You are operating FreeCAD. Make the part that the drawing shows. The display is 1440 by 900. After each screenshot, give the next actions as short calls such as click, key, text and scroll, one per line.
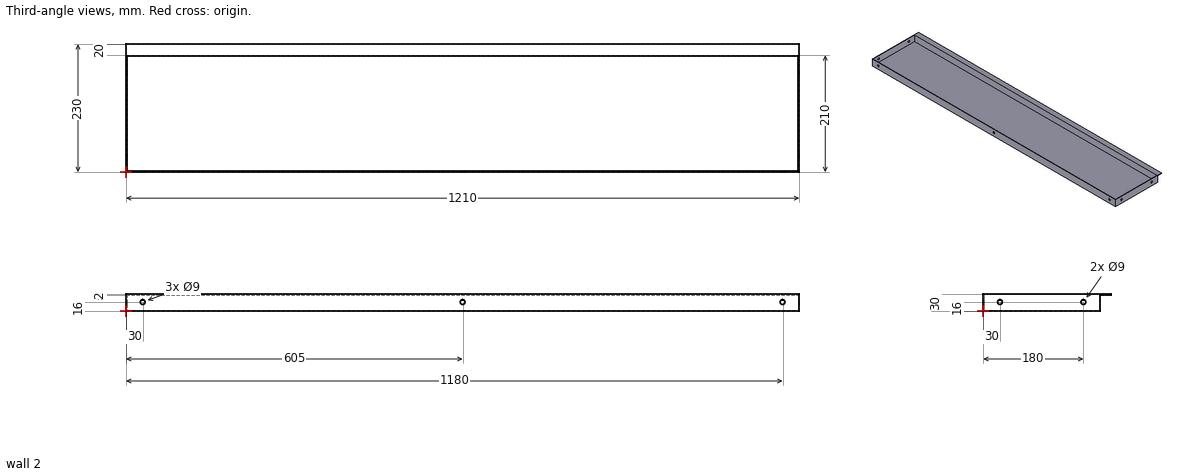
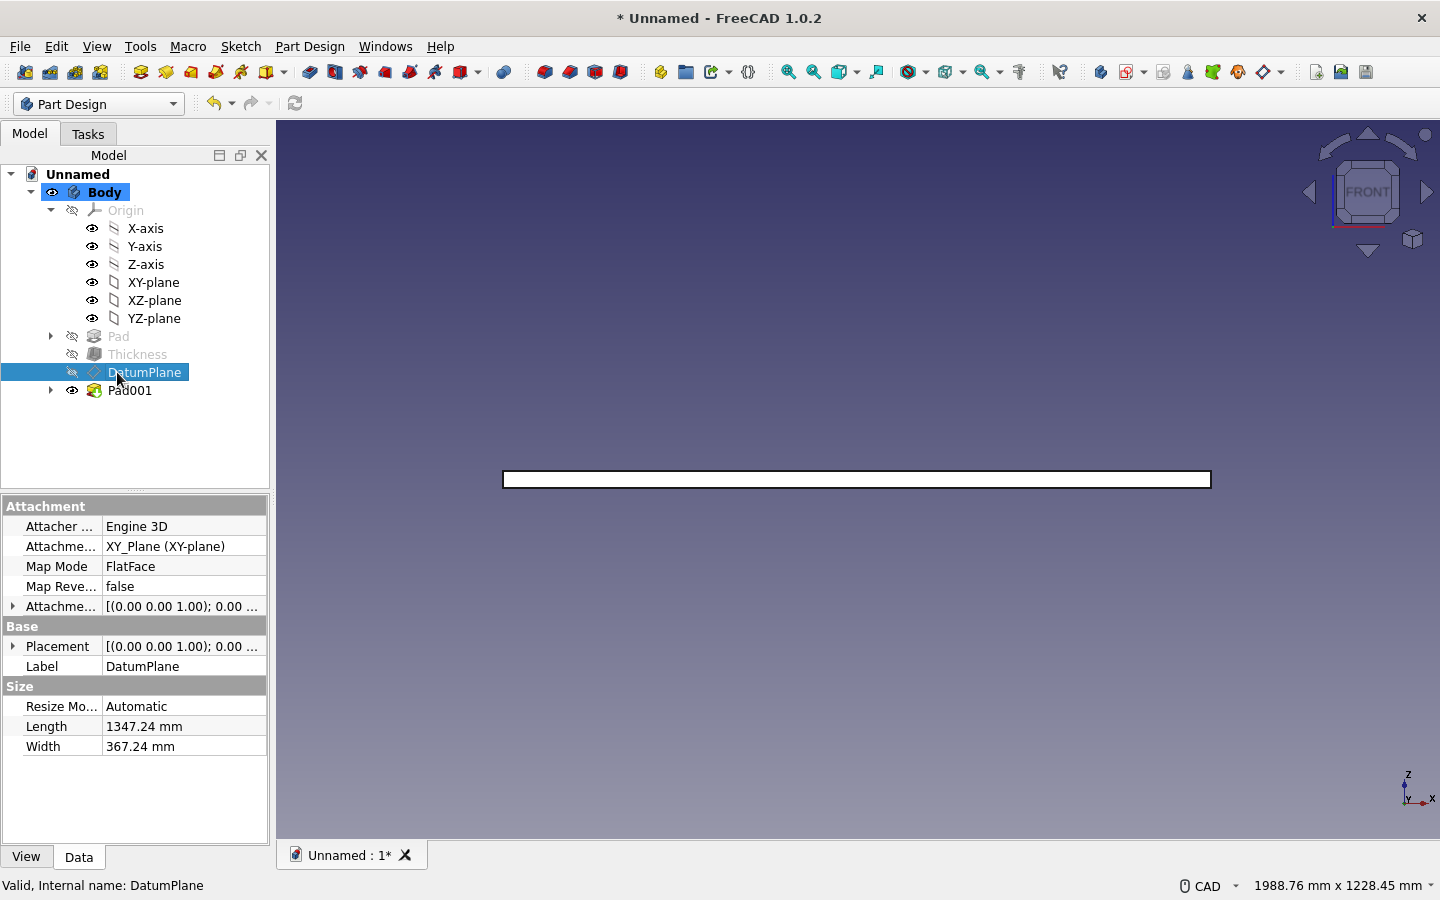
click(137, 300)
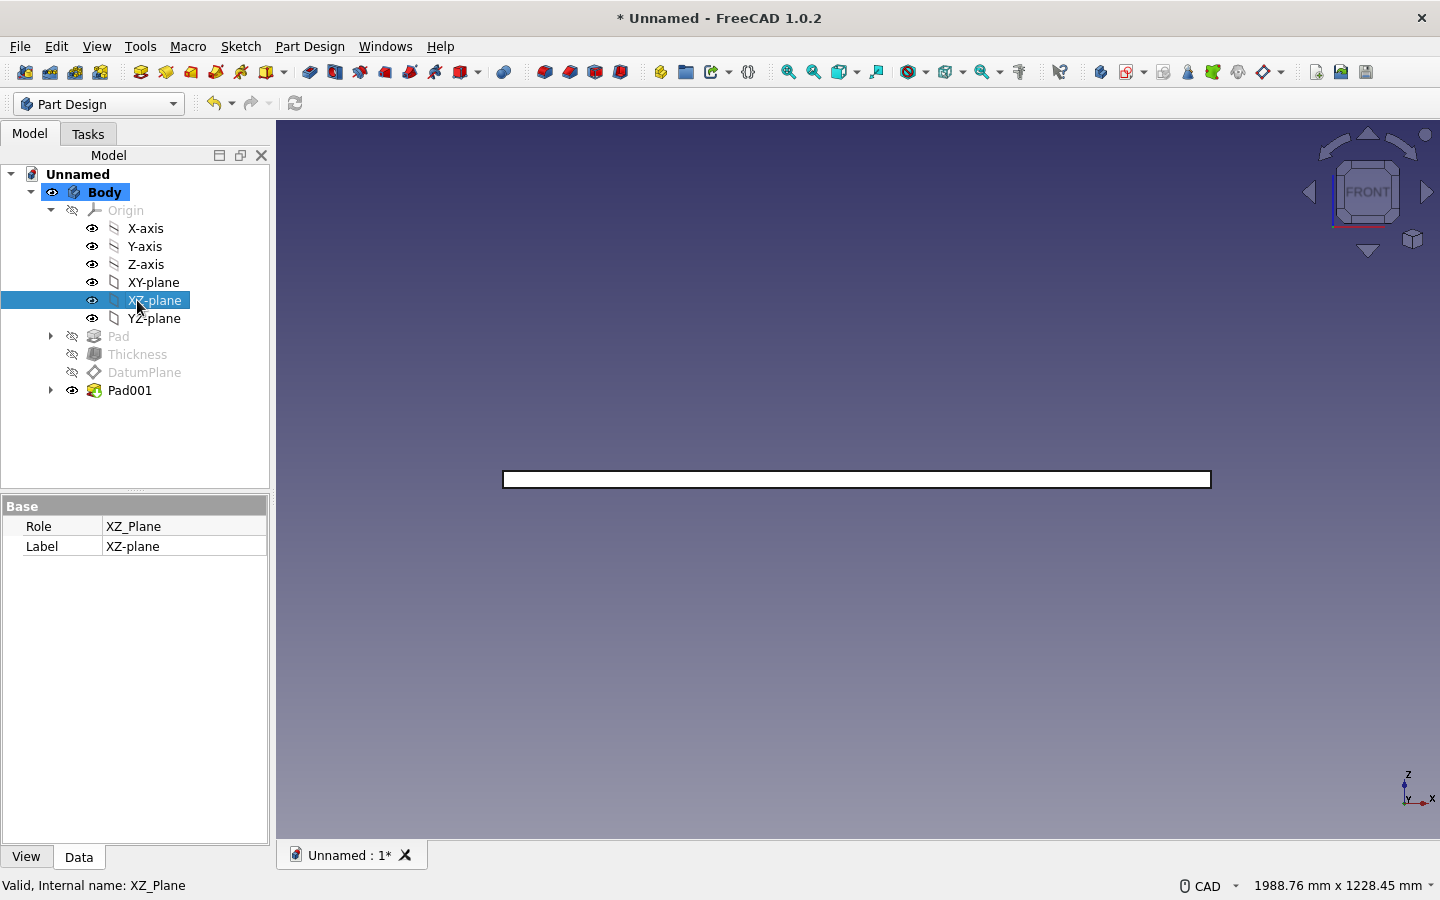
click(1262, 72)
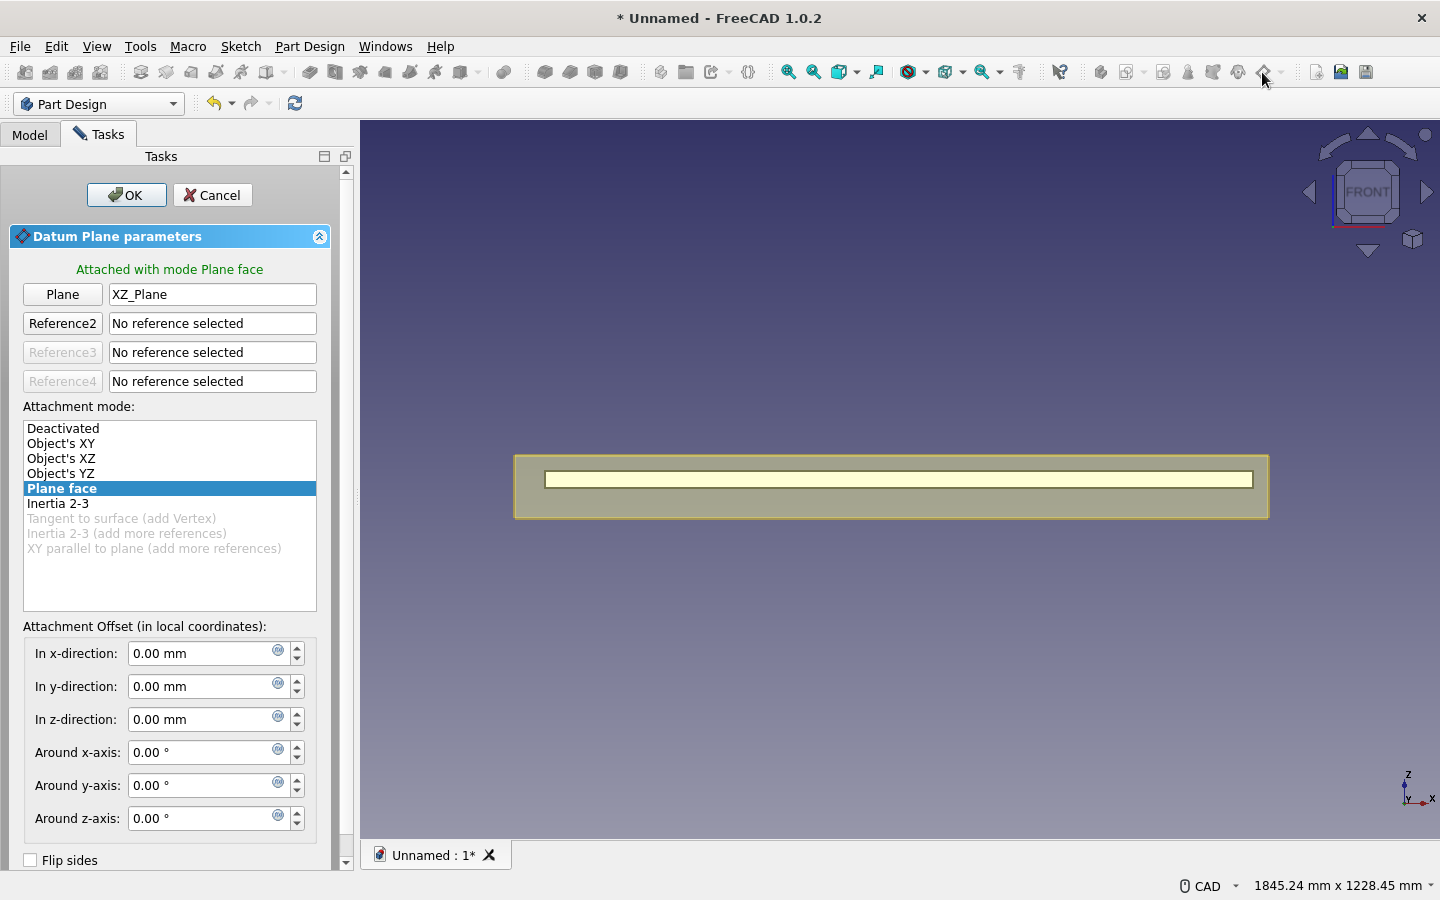
triple_click(210, 720)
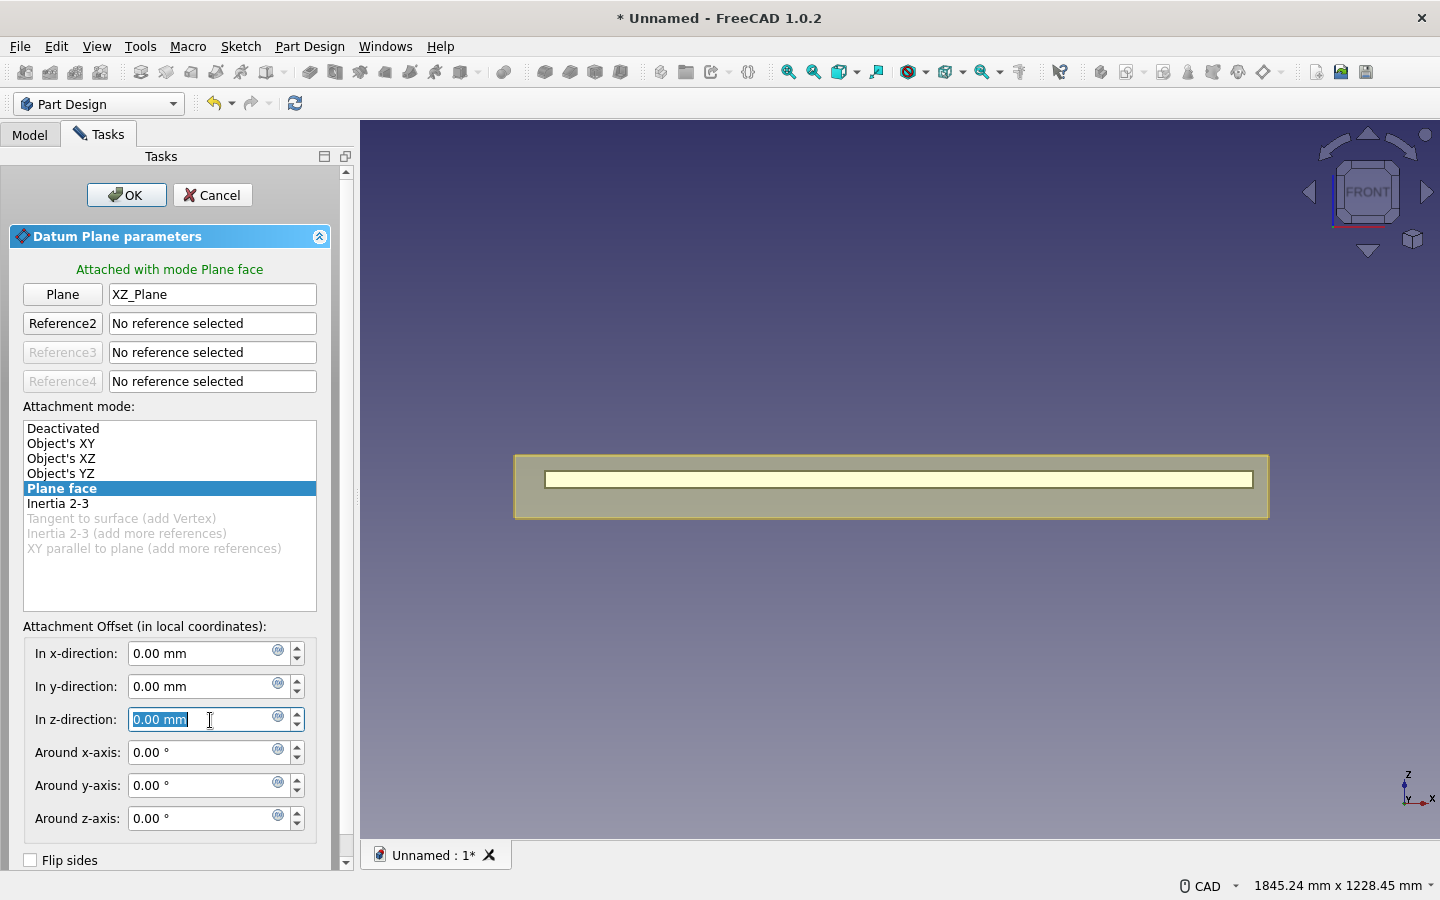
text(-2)
key(Tab)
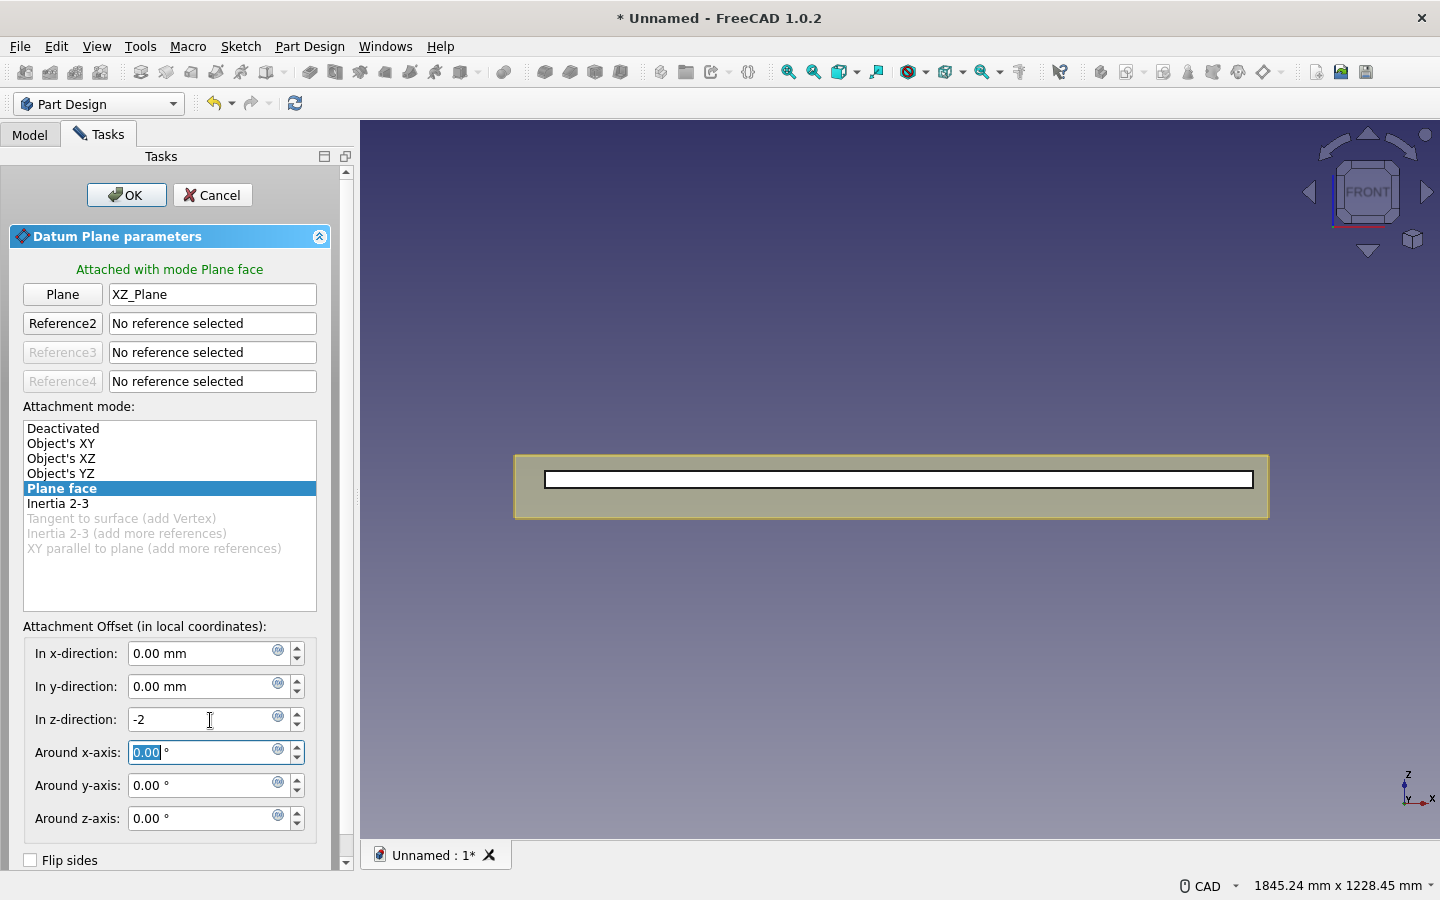
click(127, 195)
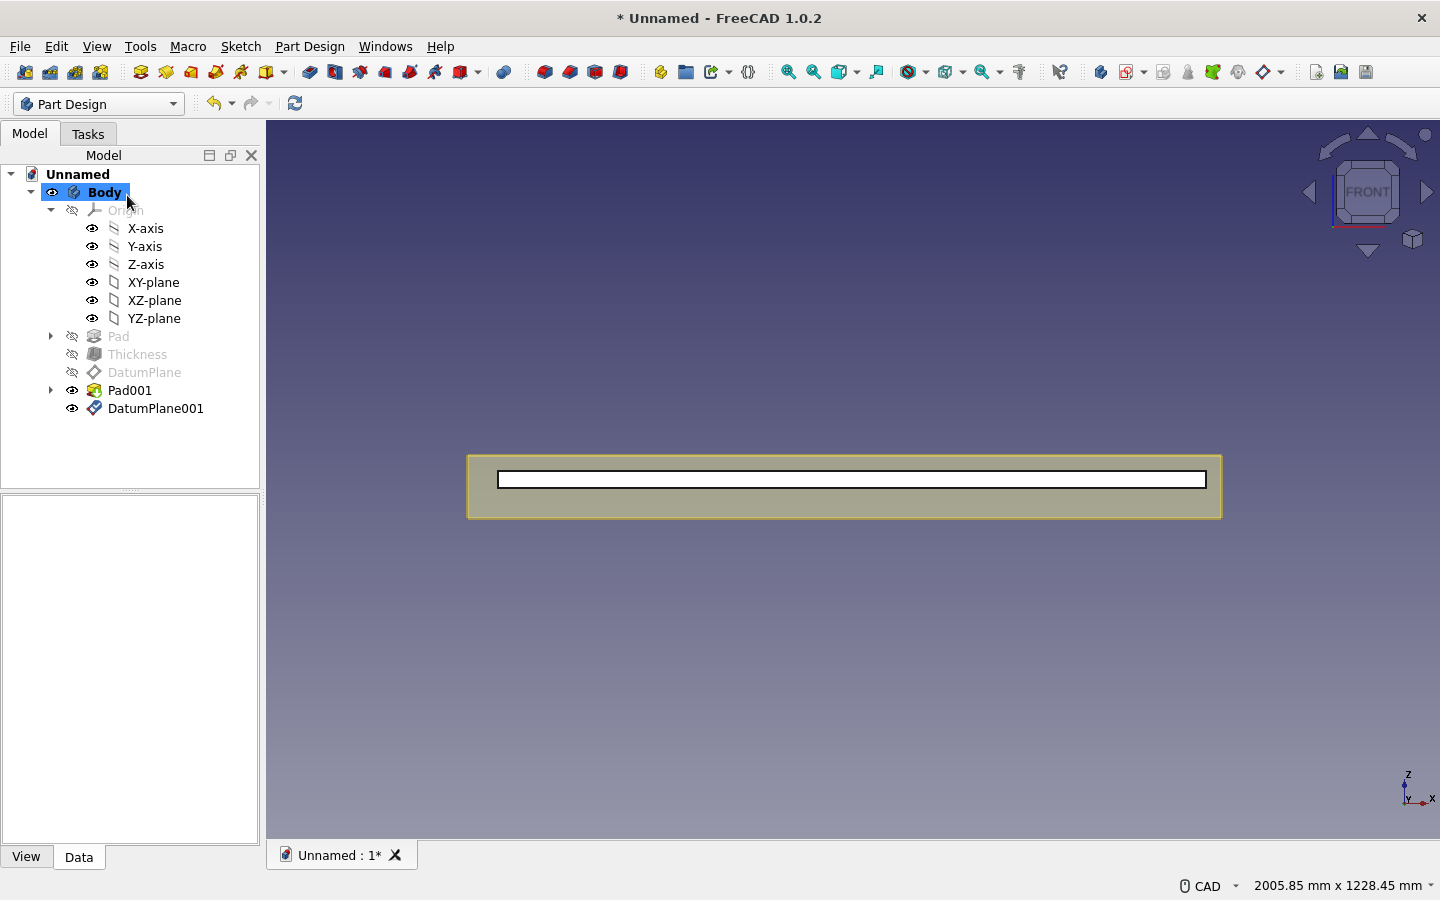
click(117, 408)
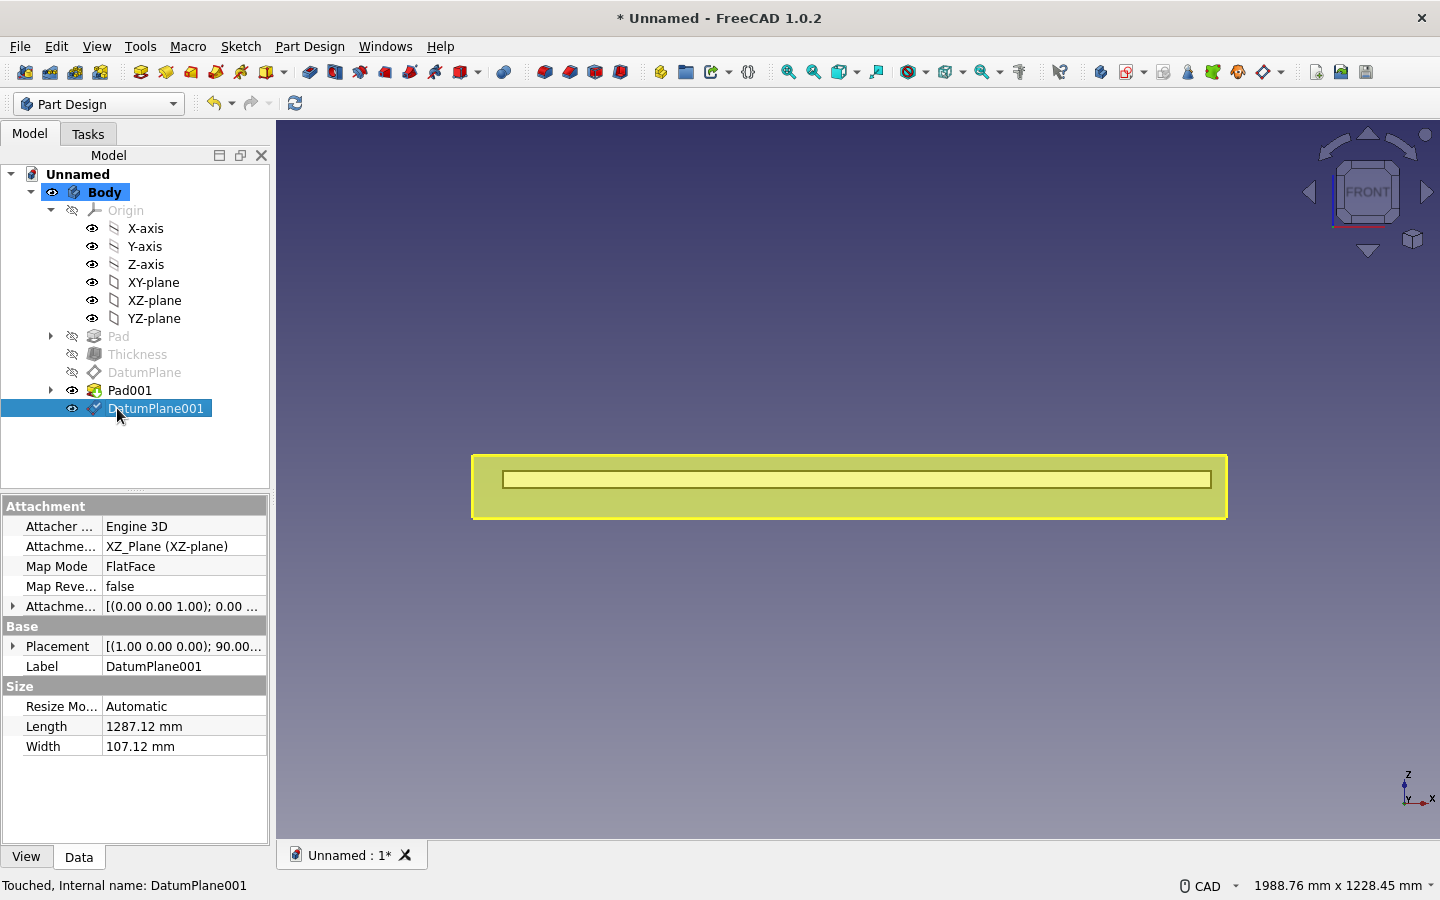
click(1126, 72)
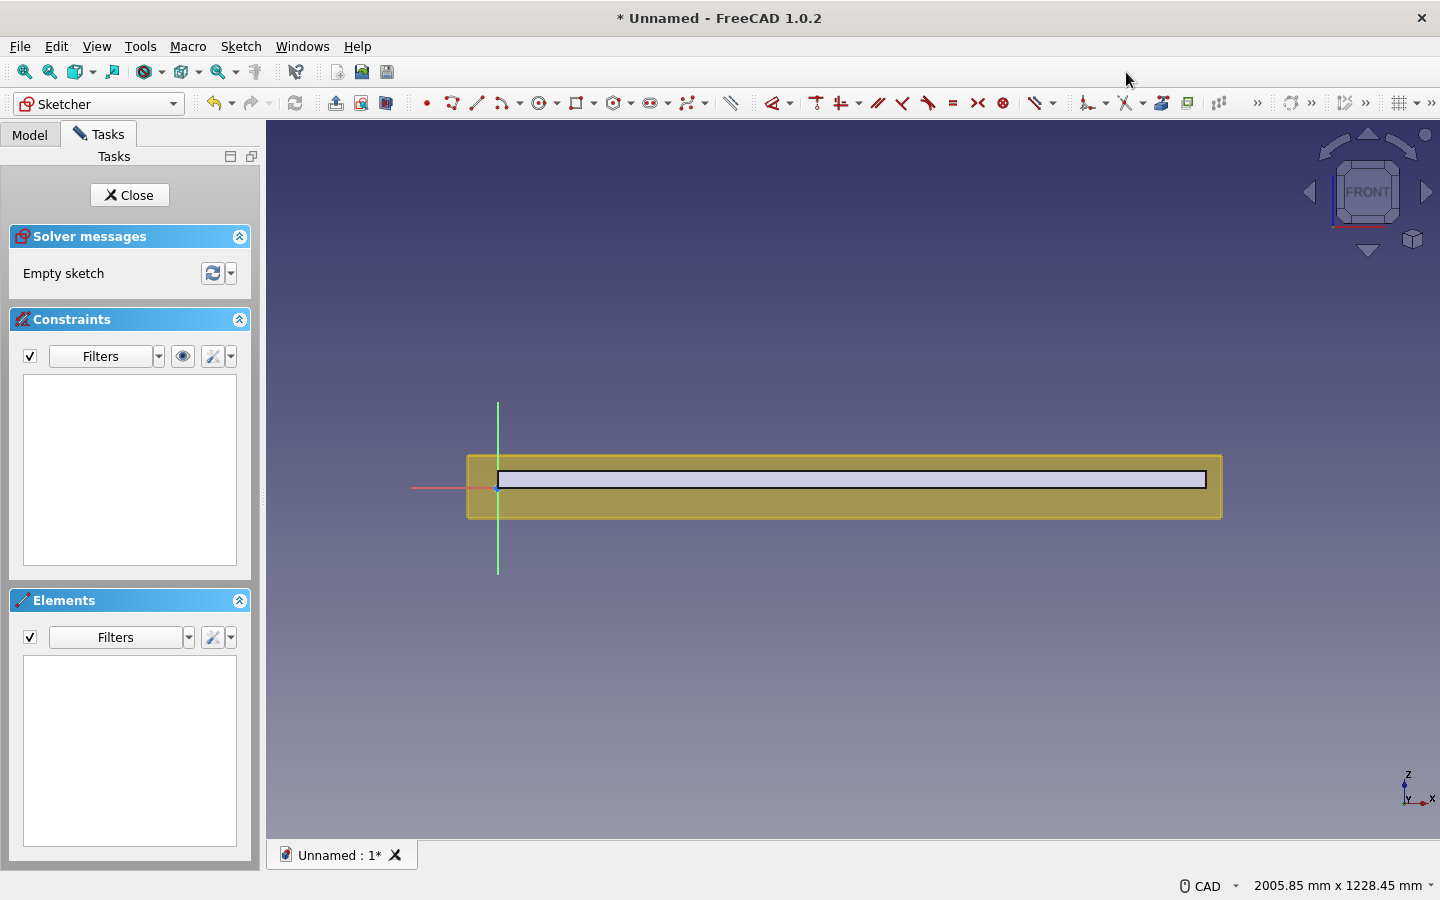
click(386, 104)